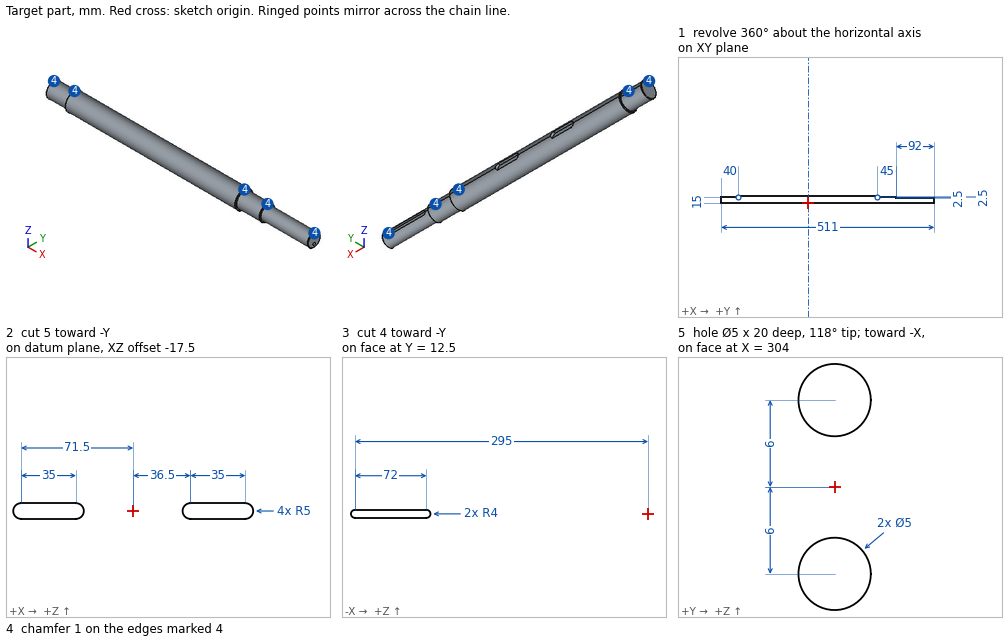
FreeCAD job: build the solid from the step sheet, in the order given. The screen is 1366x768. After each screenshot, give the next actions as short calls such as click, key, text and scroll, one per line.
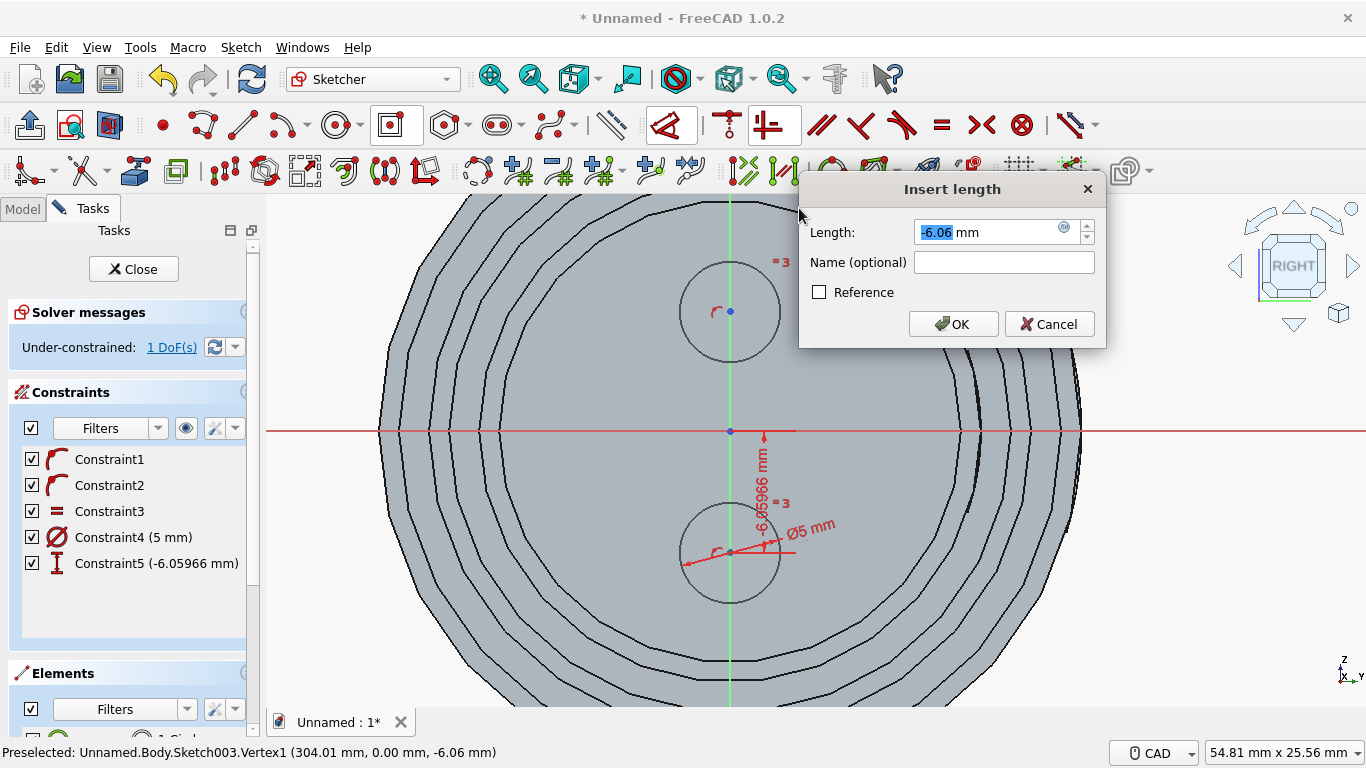
text(-6)
key(Return)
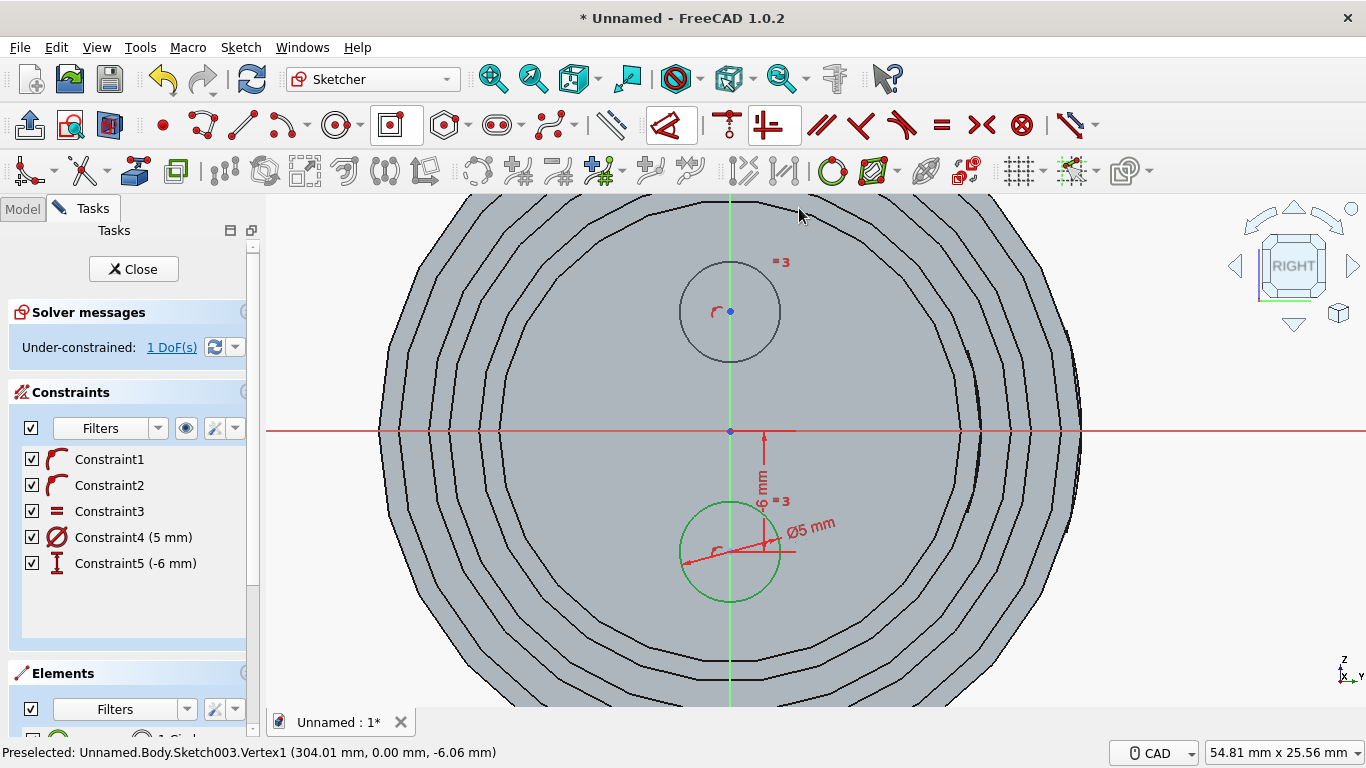
click(730, 312)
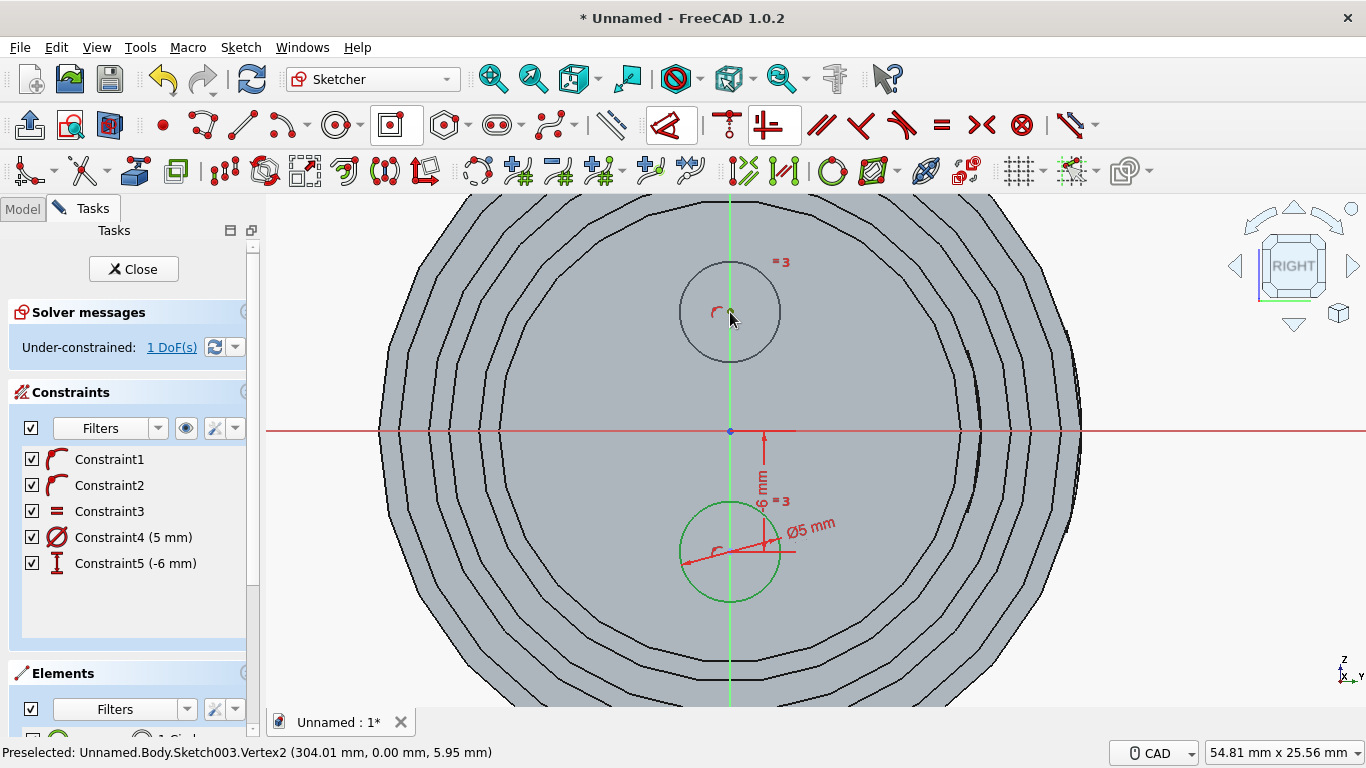
click(692, 126)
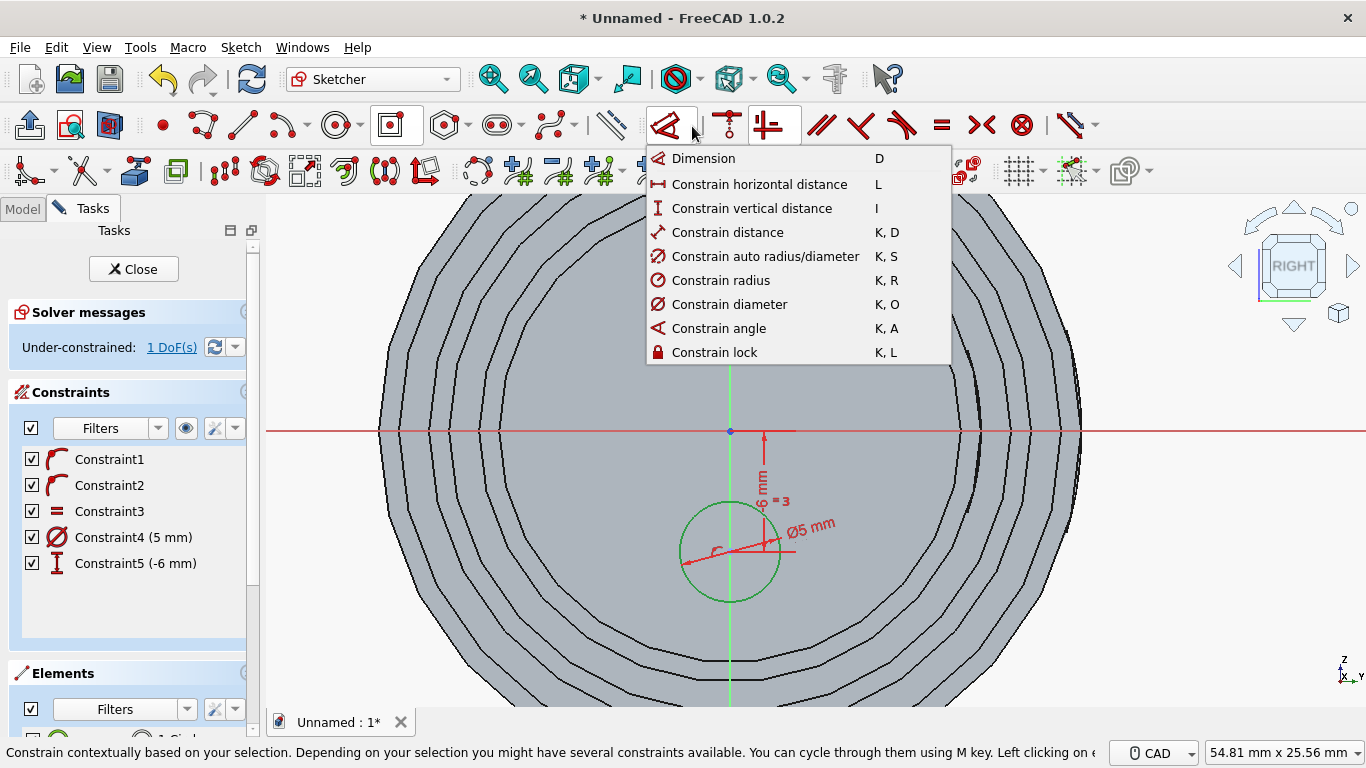
click(799, 208)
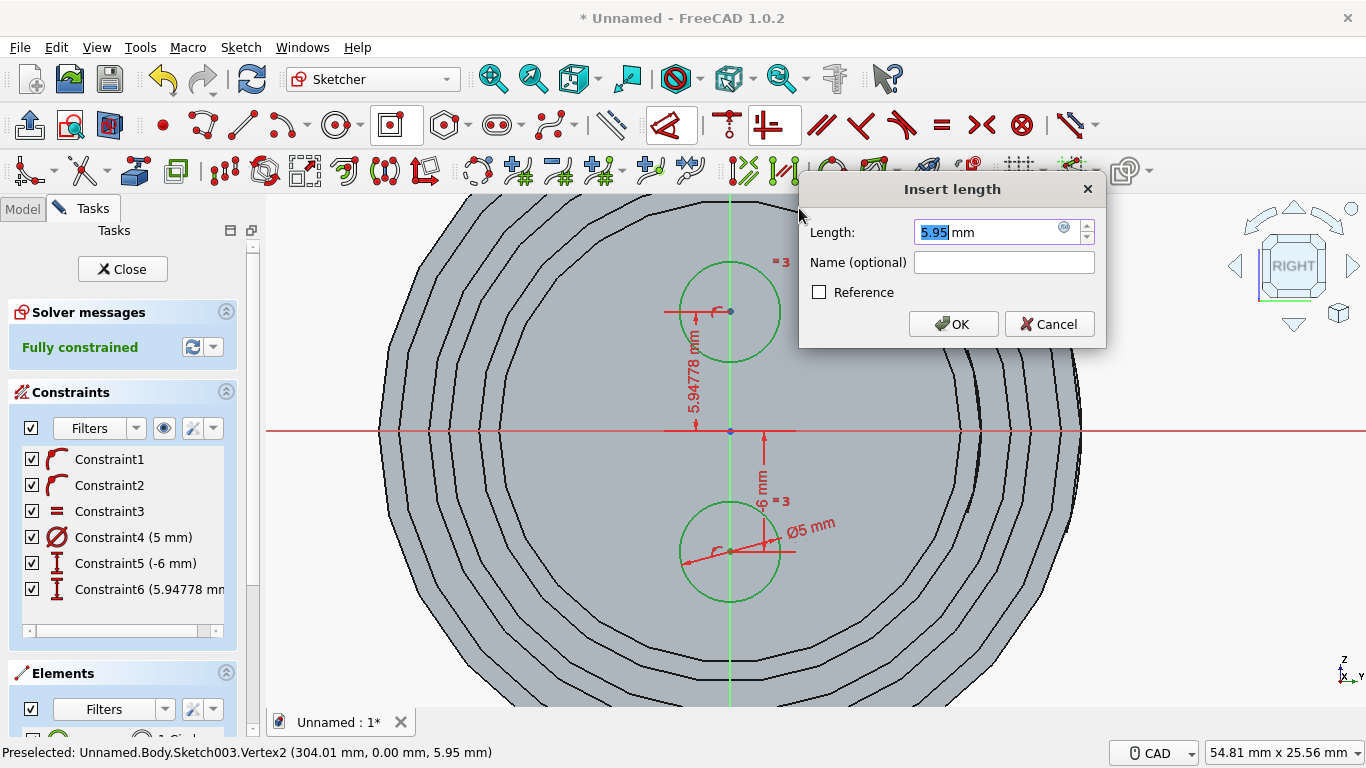
text(6)
key(Return)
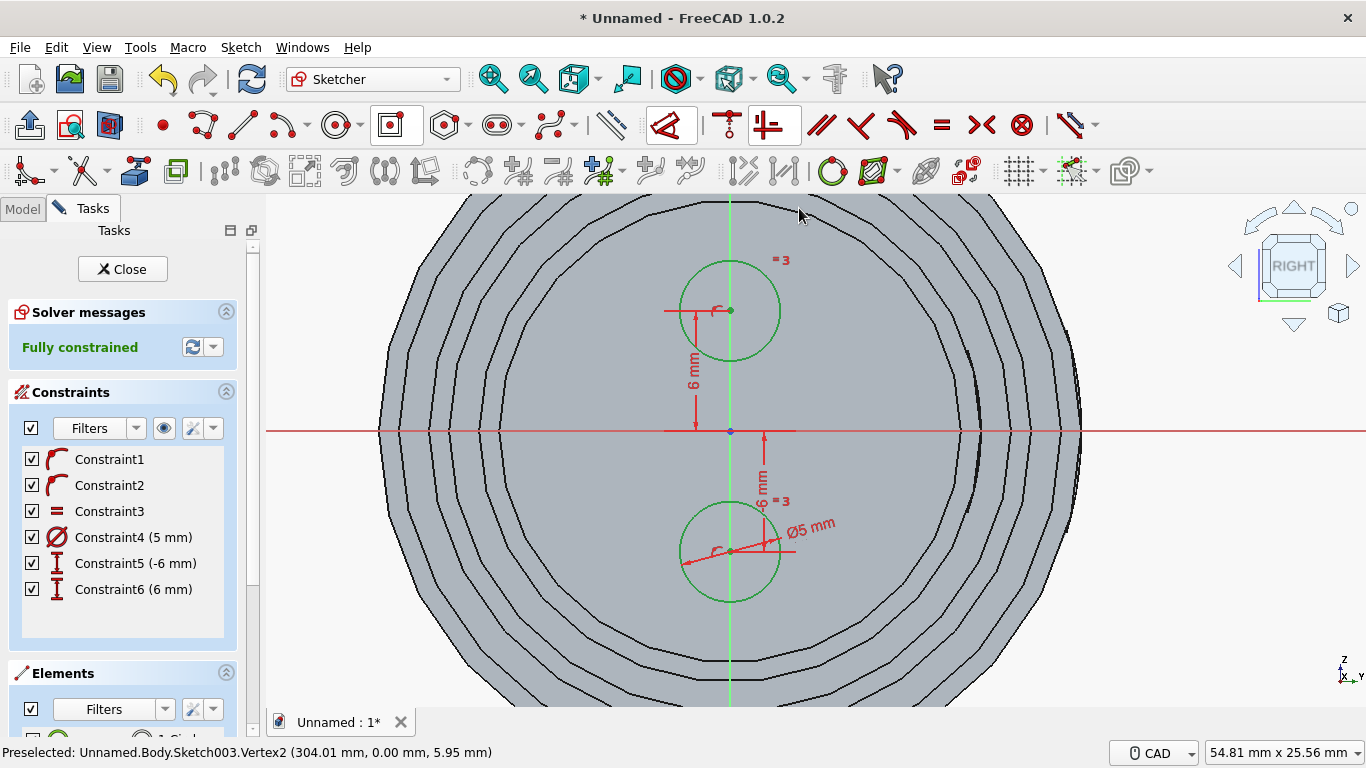
click(123, 269)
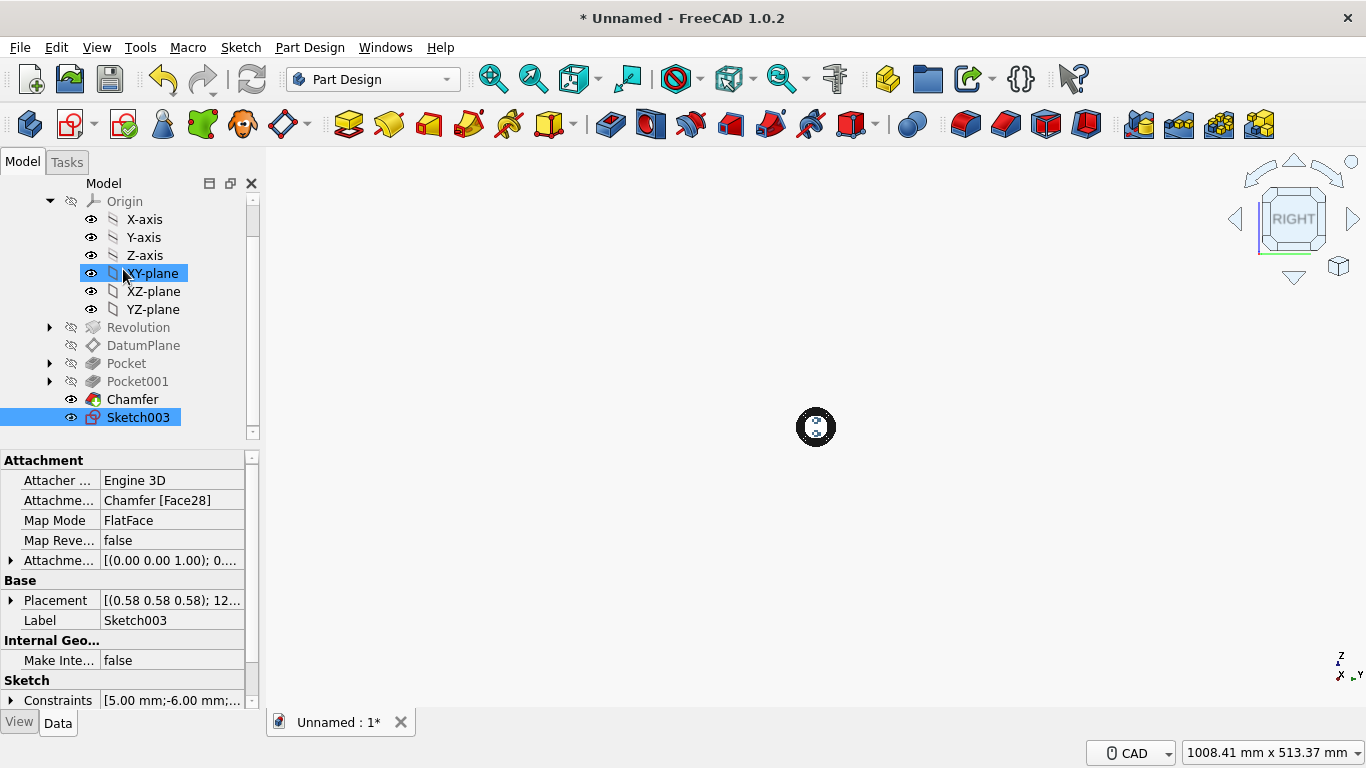
click(652, 124)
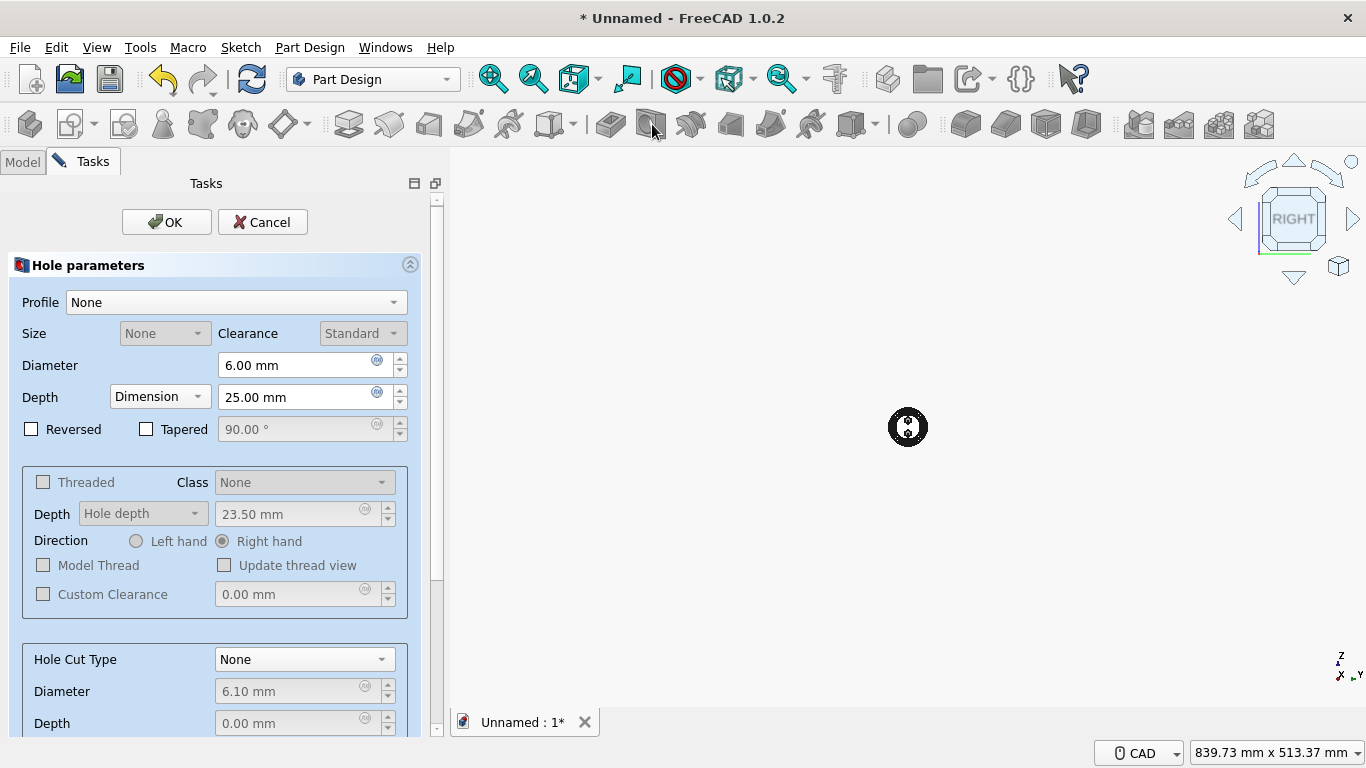
triple_click(305, 365)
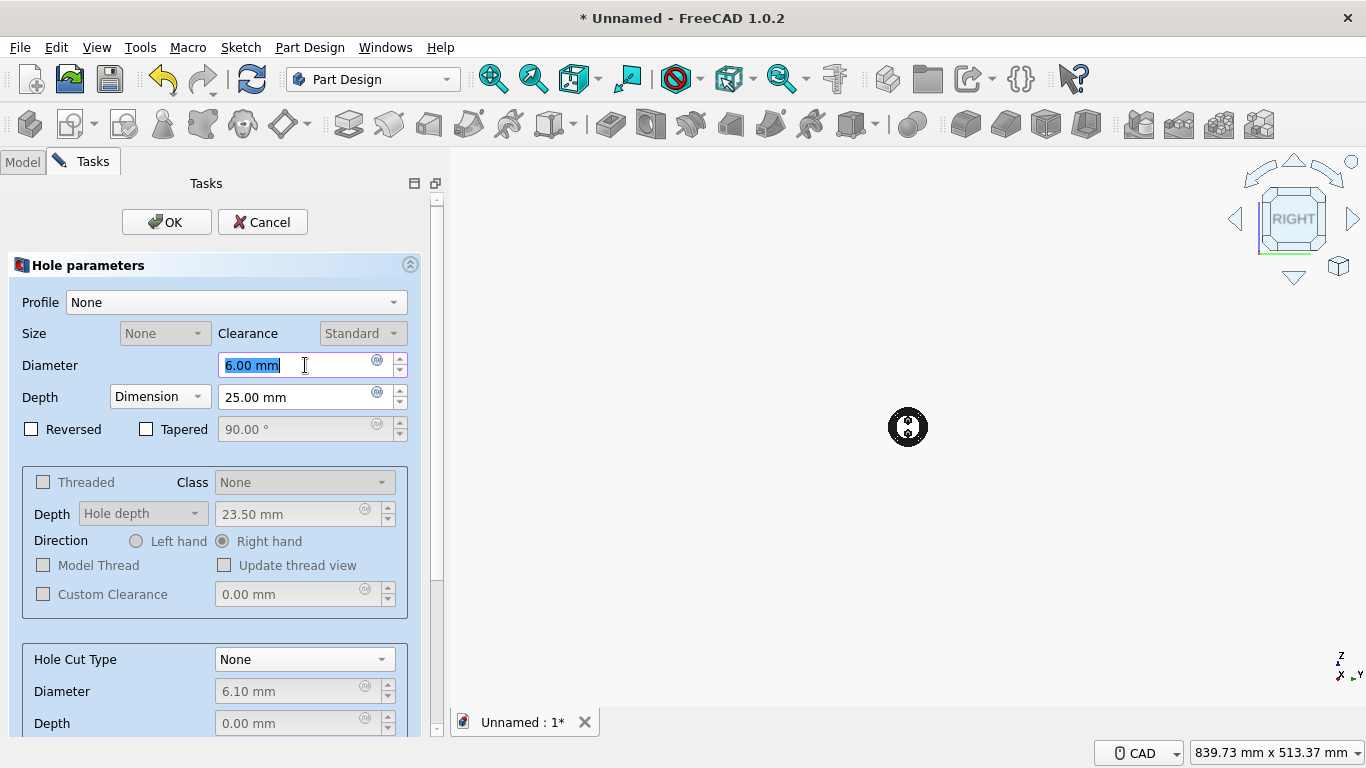
text(5)
key(Tab)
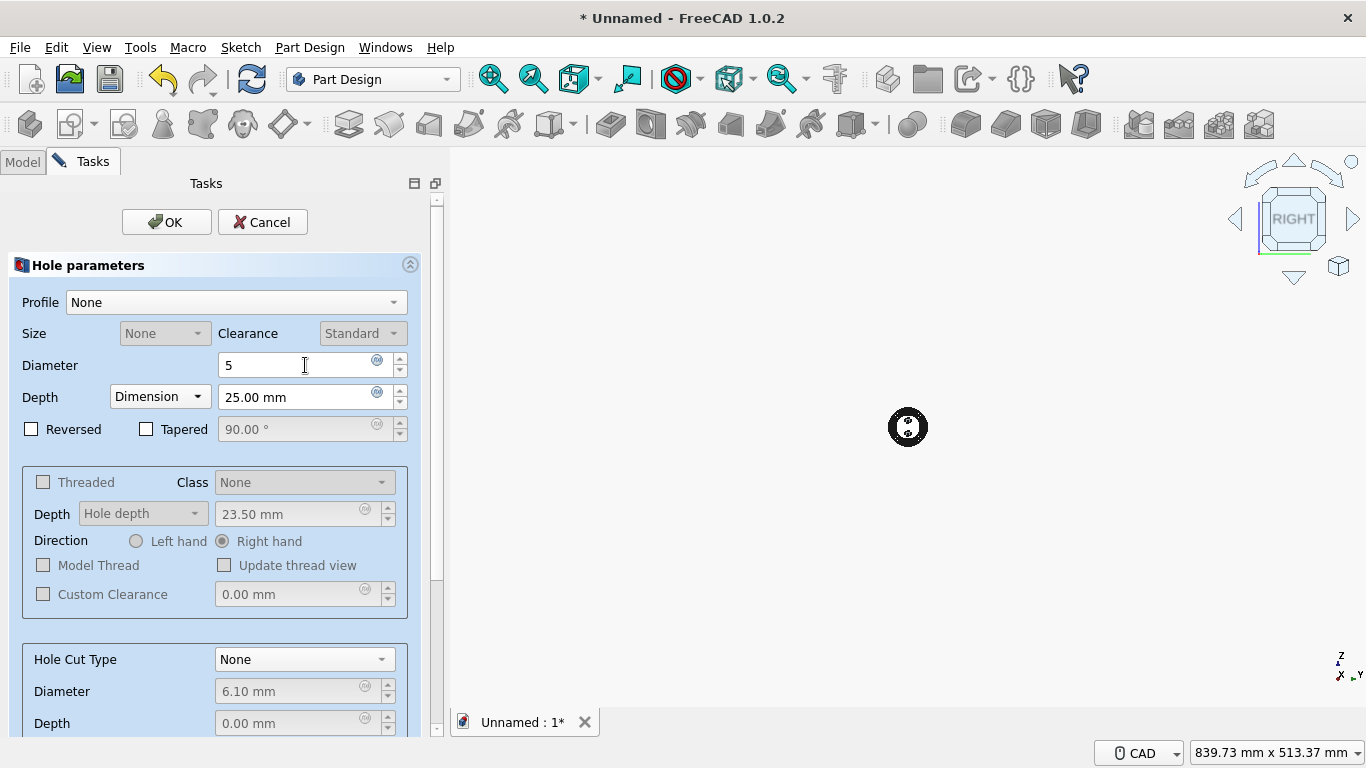
triple_click(305, 397)